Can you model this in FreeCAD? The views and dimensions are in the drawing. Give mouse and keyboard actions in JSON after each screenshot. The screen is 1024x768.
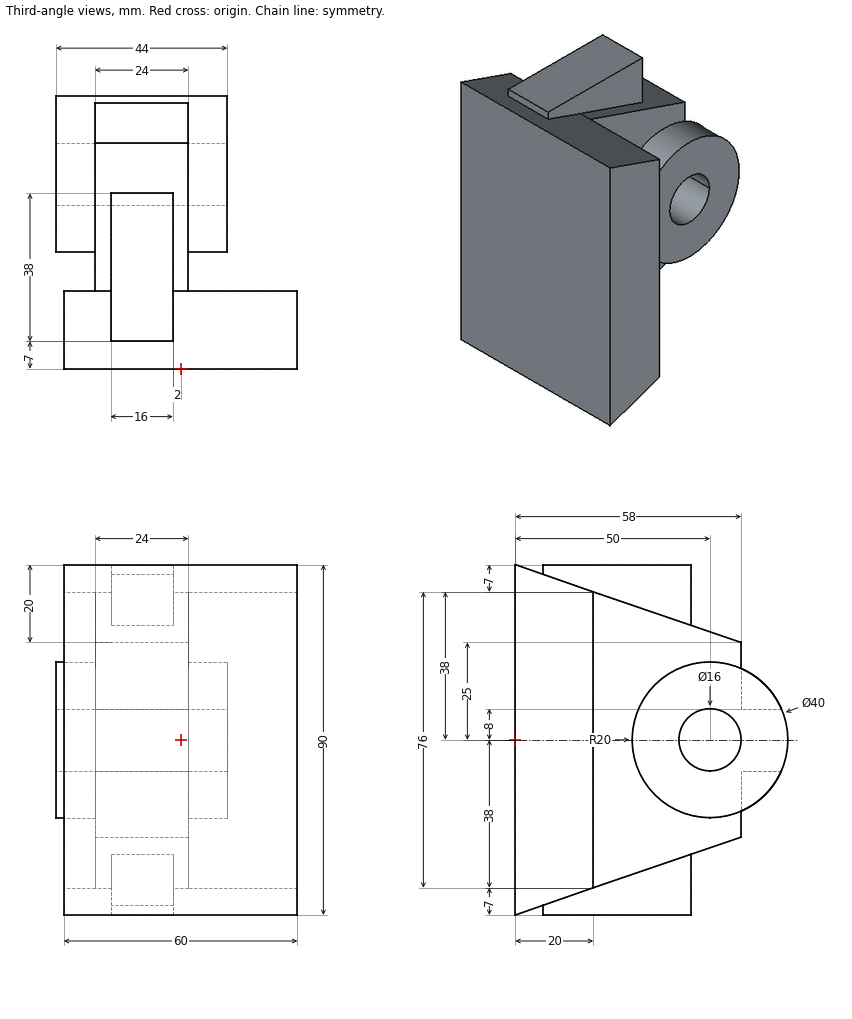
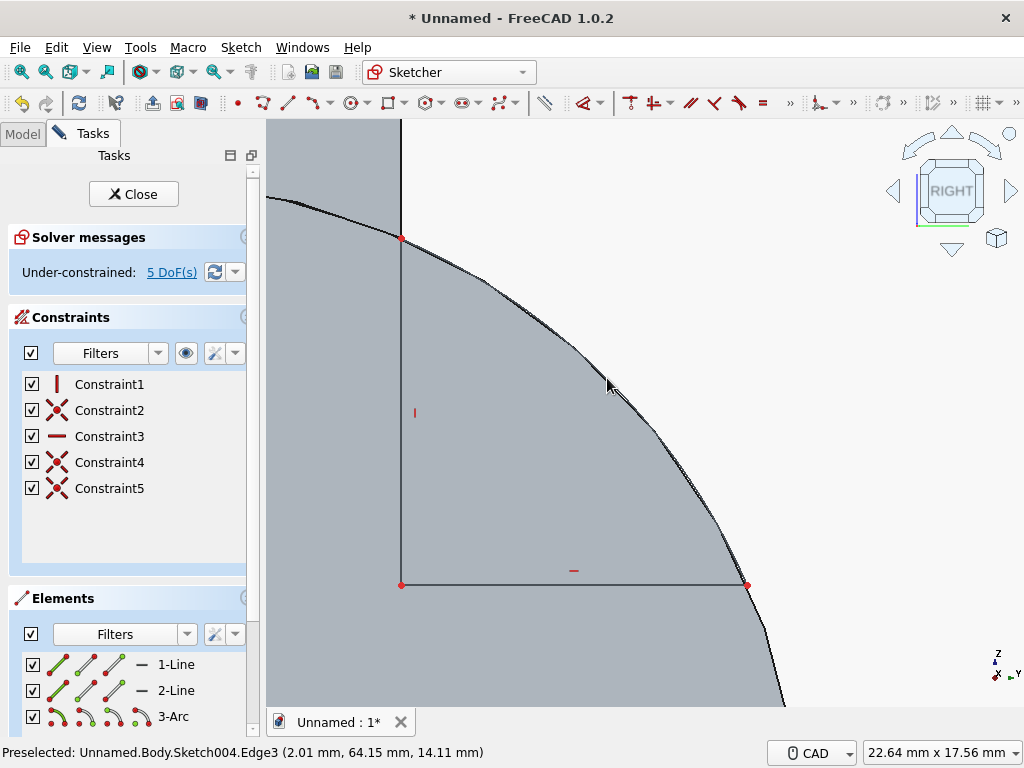
{"action": "scroll", "coordinate": [850, 148], "scroll_direction": "down", "scroll_amount": 2}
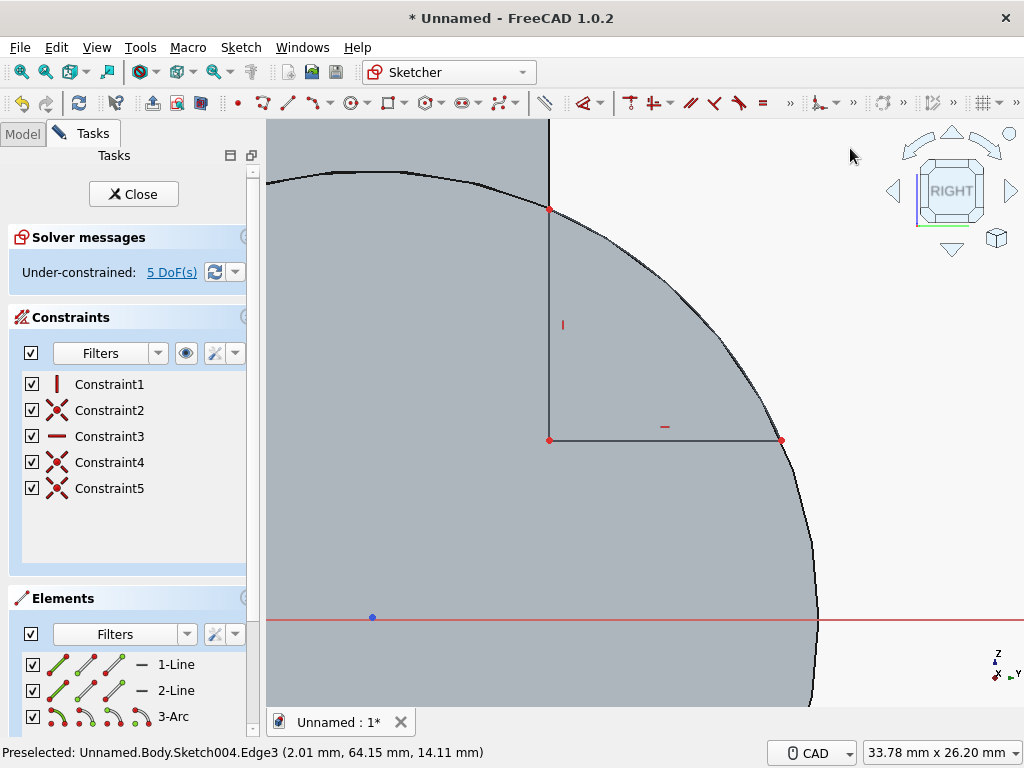
{"action": "left_click", "coordinate": [372, 618]}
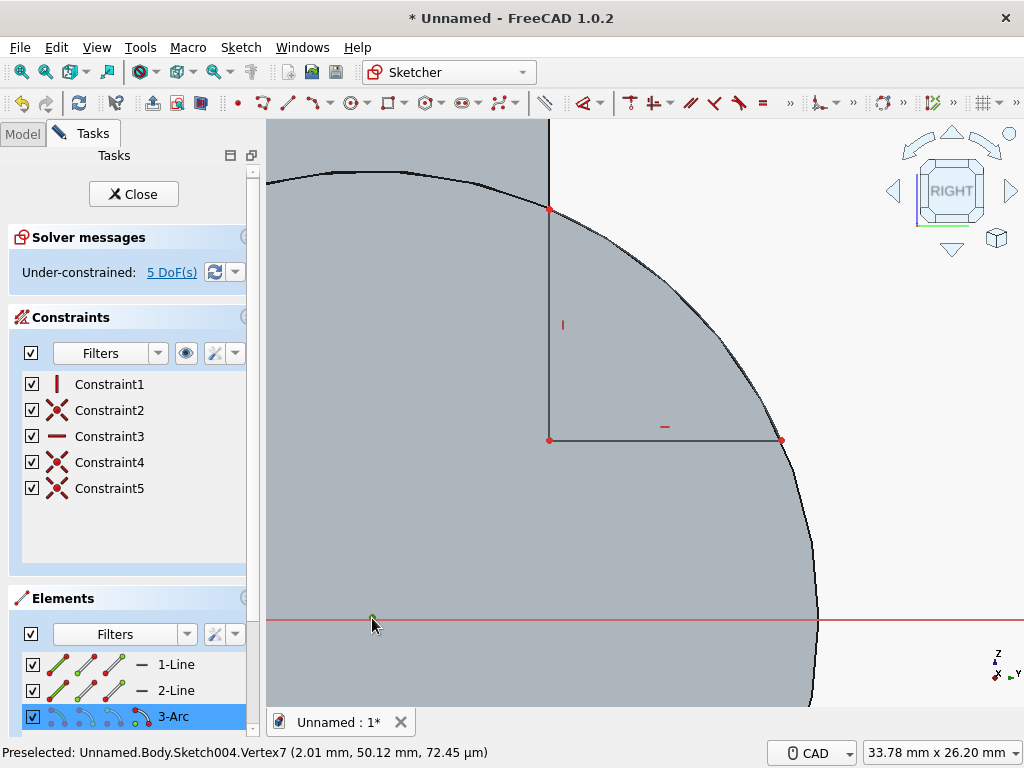
{"action": "left_click", "coordinate": [334, 620]}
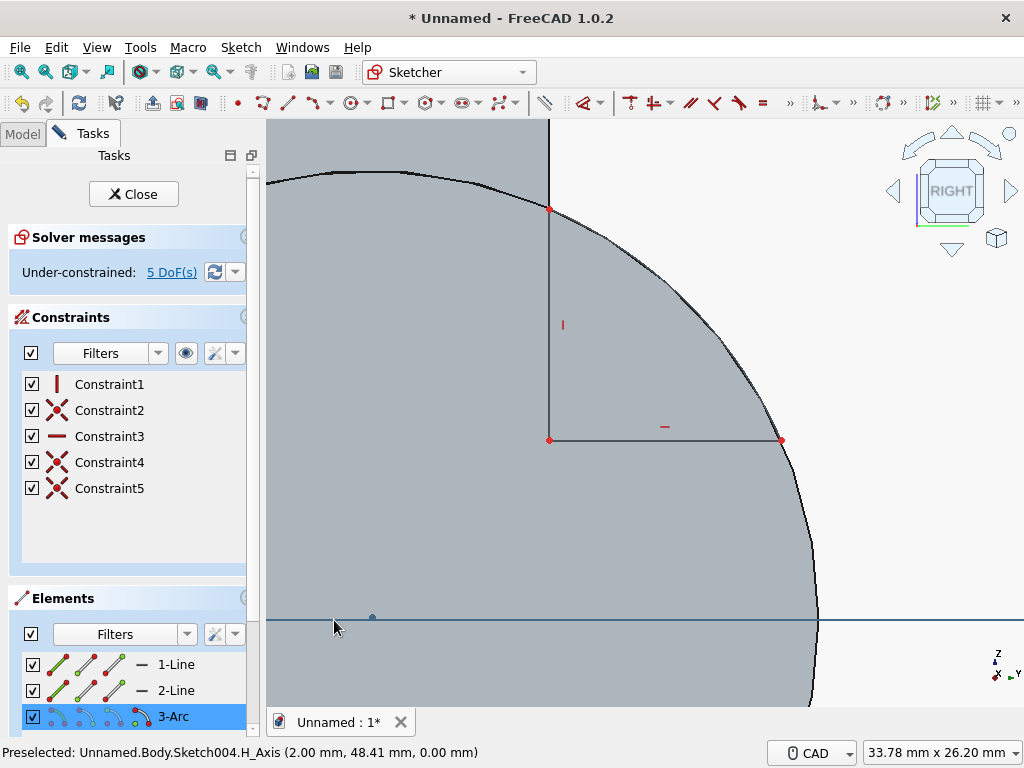
{"action": "key", "text": "c"}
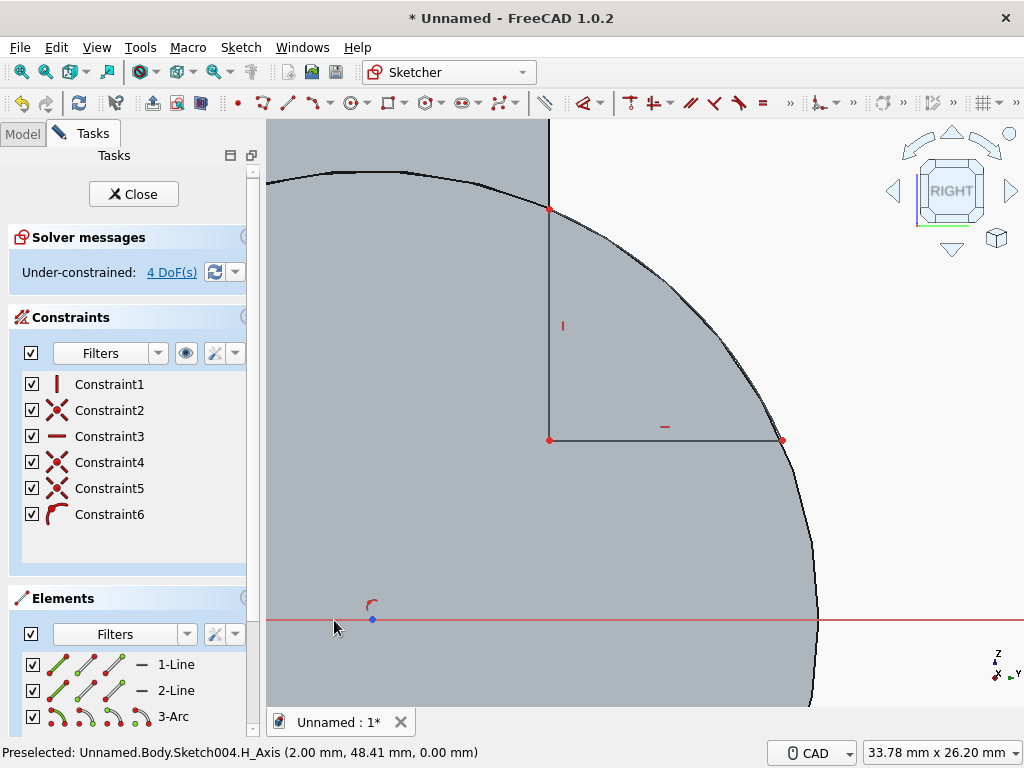
{"action": "left_click", "coordinate": [584, 104]}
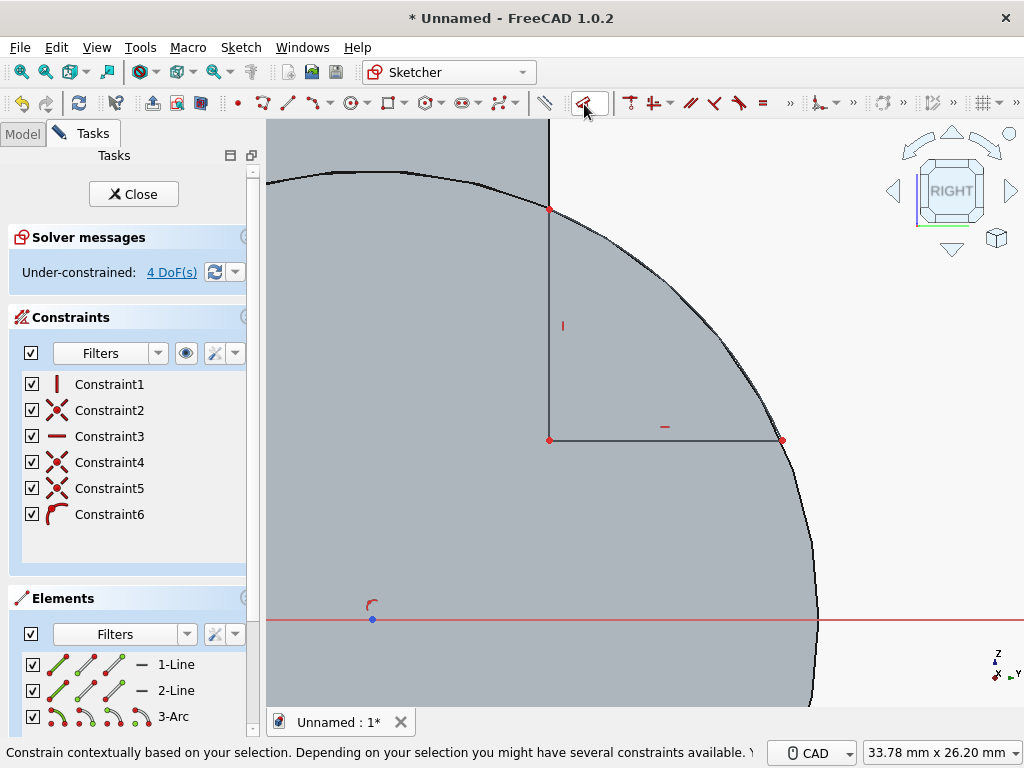
{"action": "left_click", "coordinate": [732, 354]}
{"action": "left_click", "coordinate": [758, 335]}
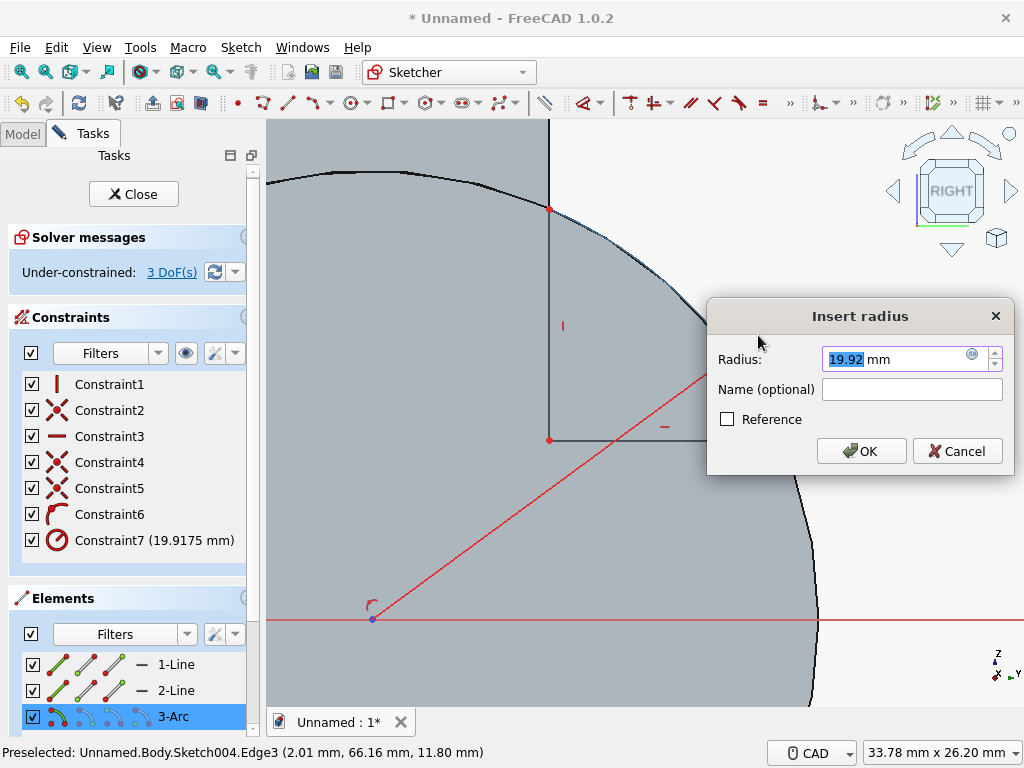
{"action": "type", "text": "20"}
{"action": "key", "text": "Return"}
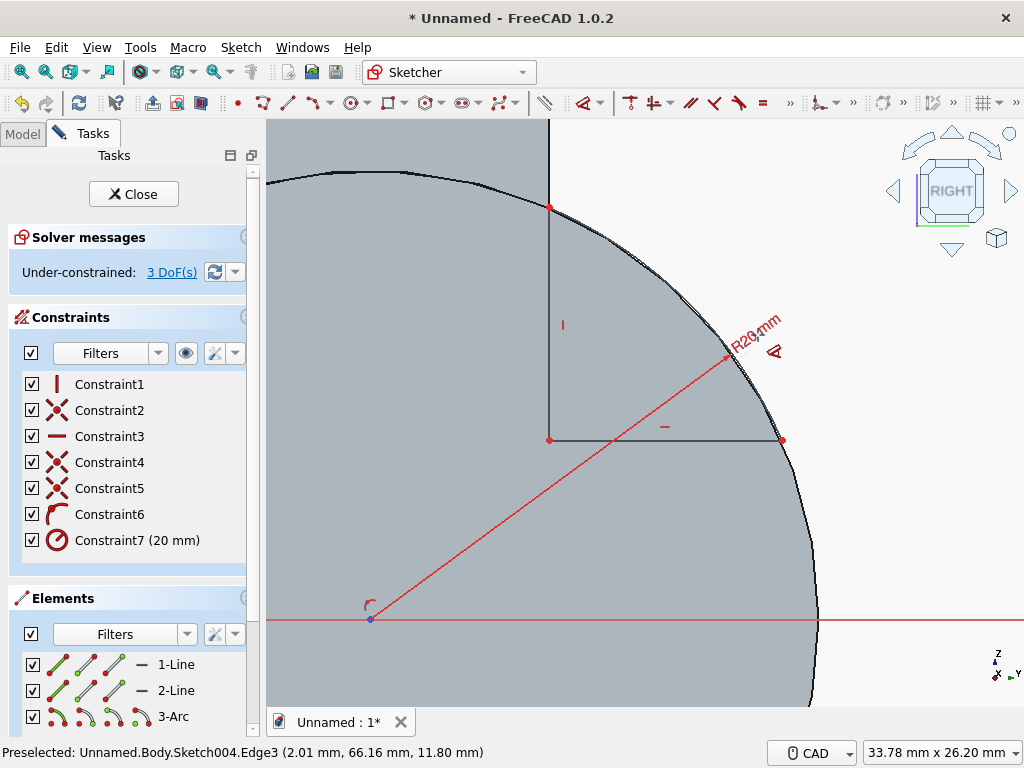
{"action": "left_click", "coordinate": [549, 441]}
{"action": "left_click", "coordinate": [583, 530]}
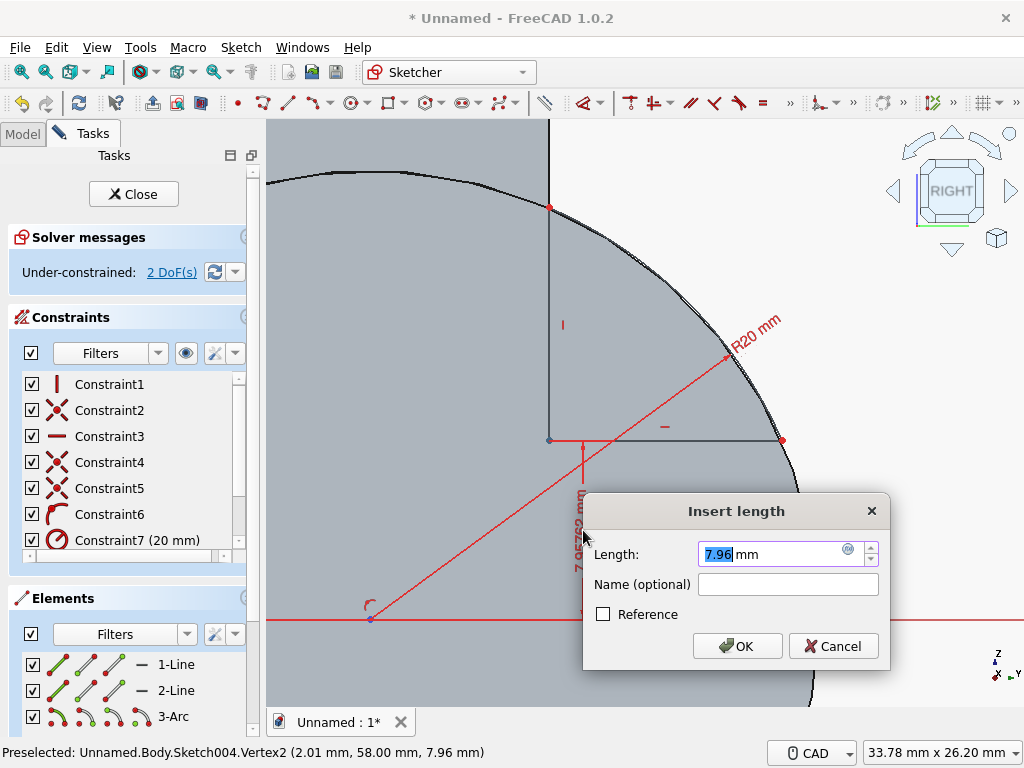
{"action": "type", "text": "8"}
{"action": "key", "text": "Return"}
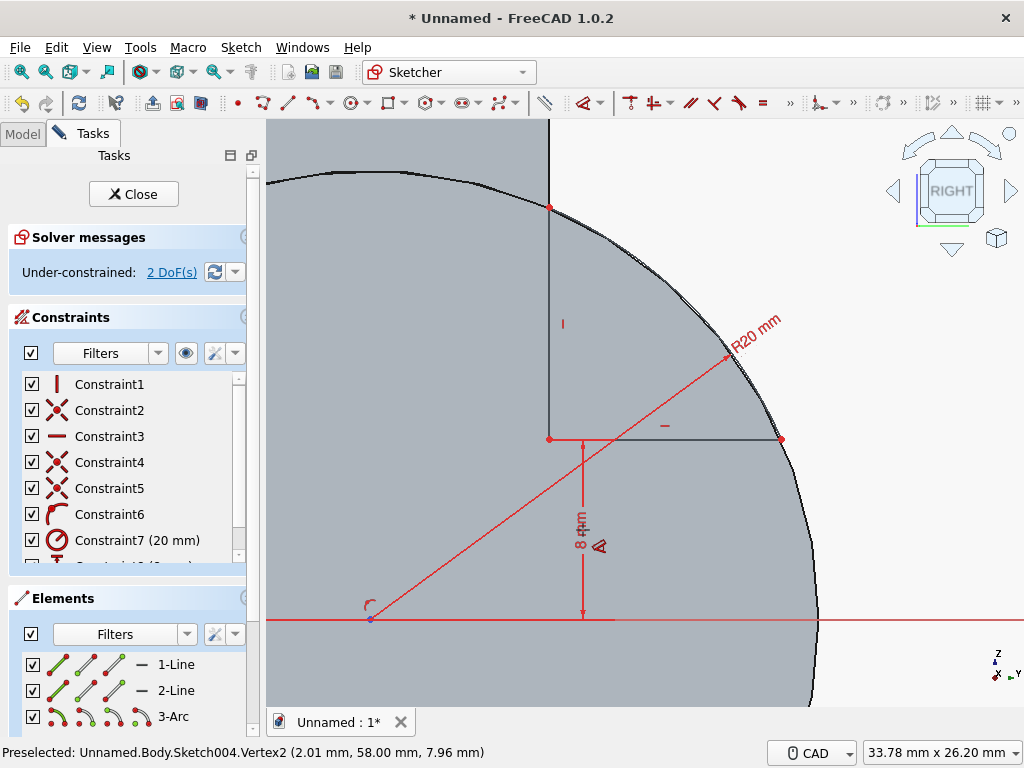
{"action": "left_click", "coordinate": [549, 208]}
{"action": "left_click", "coordinate": [422, 654]}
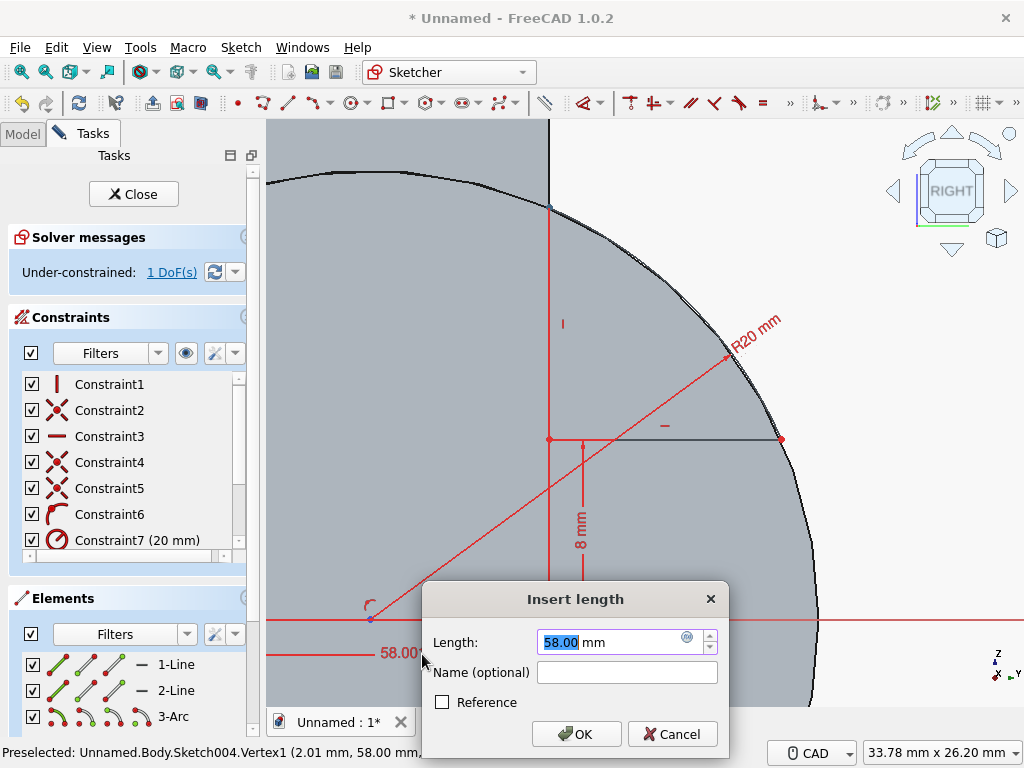
{"action": "type", "text": "58"}
{"action": "key", "text": "Return"}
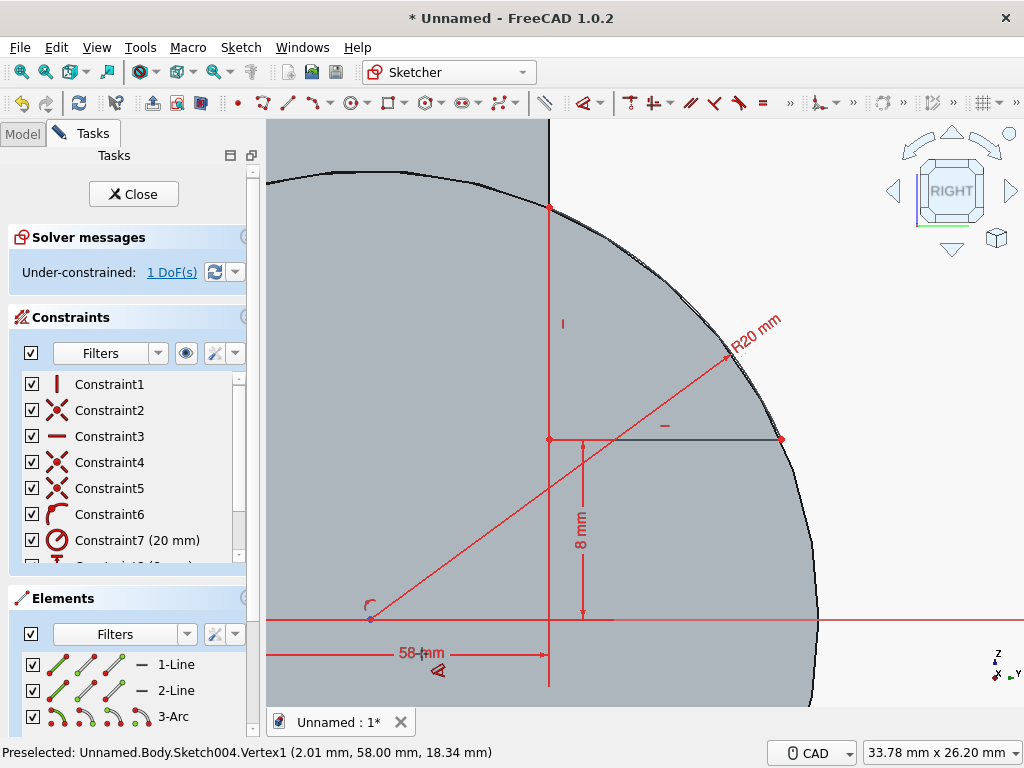
{"action": "left_click", "coordinate": [370, 620]}
{"action": "left_click", "coordinate": [332, 654]}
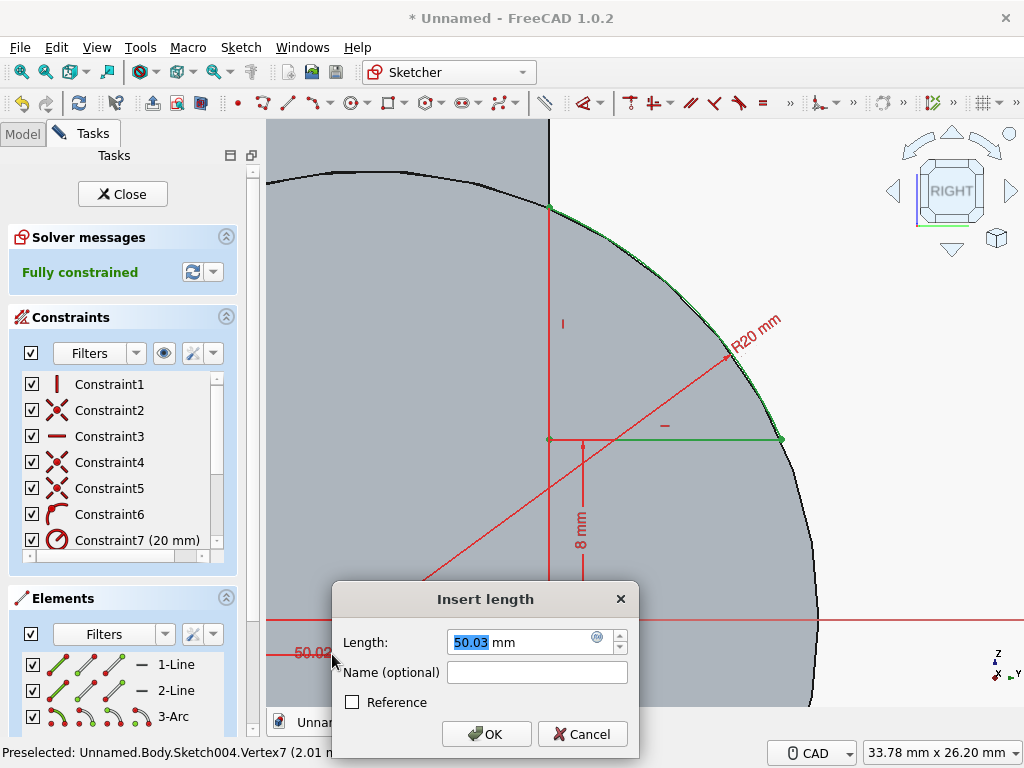
{"action": "type", "text": "50"}
{"action": "key", "text": "Return"}
{"action": "key", "text": "Escape"}